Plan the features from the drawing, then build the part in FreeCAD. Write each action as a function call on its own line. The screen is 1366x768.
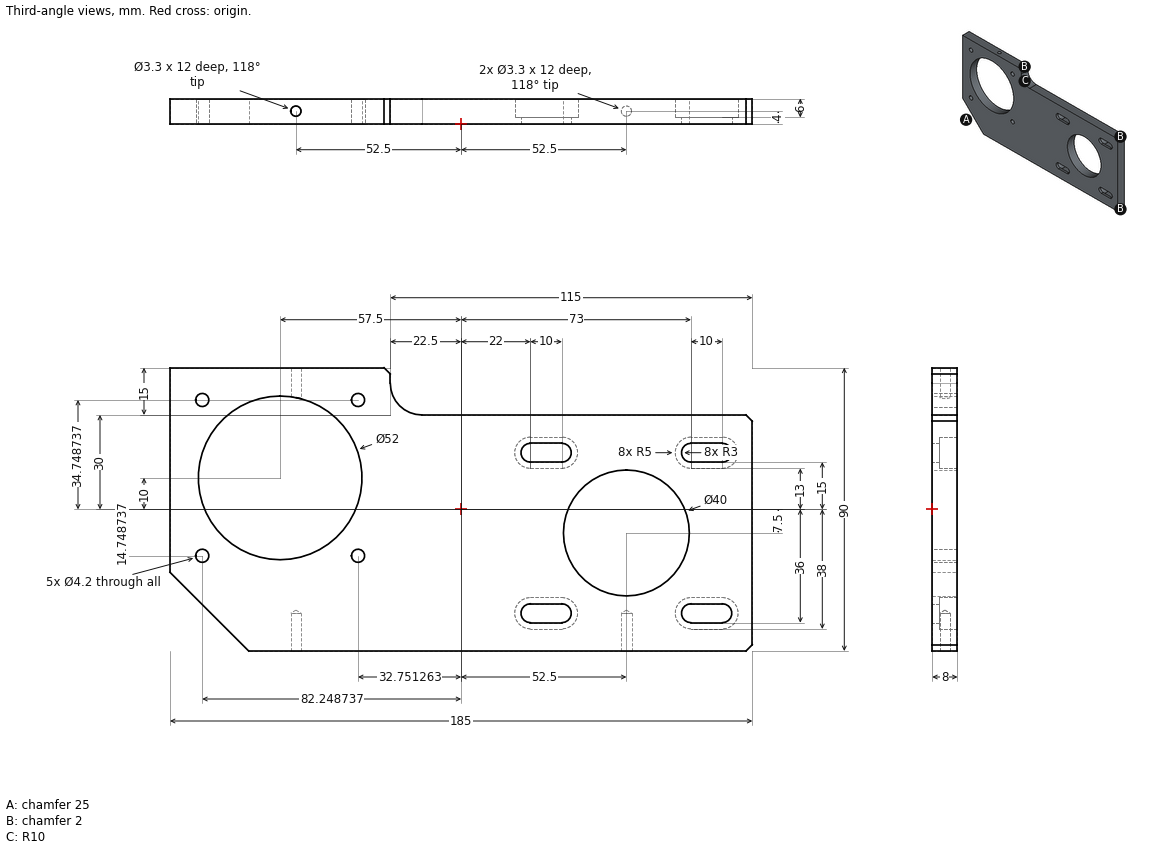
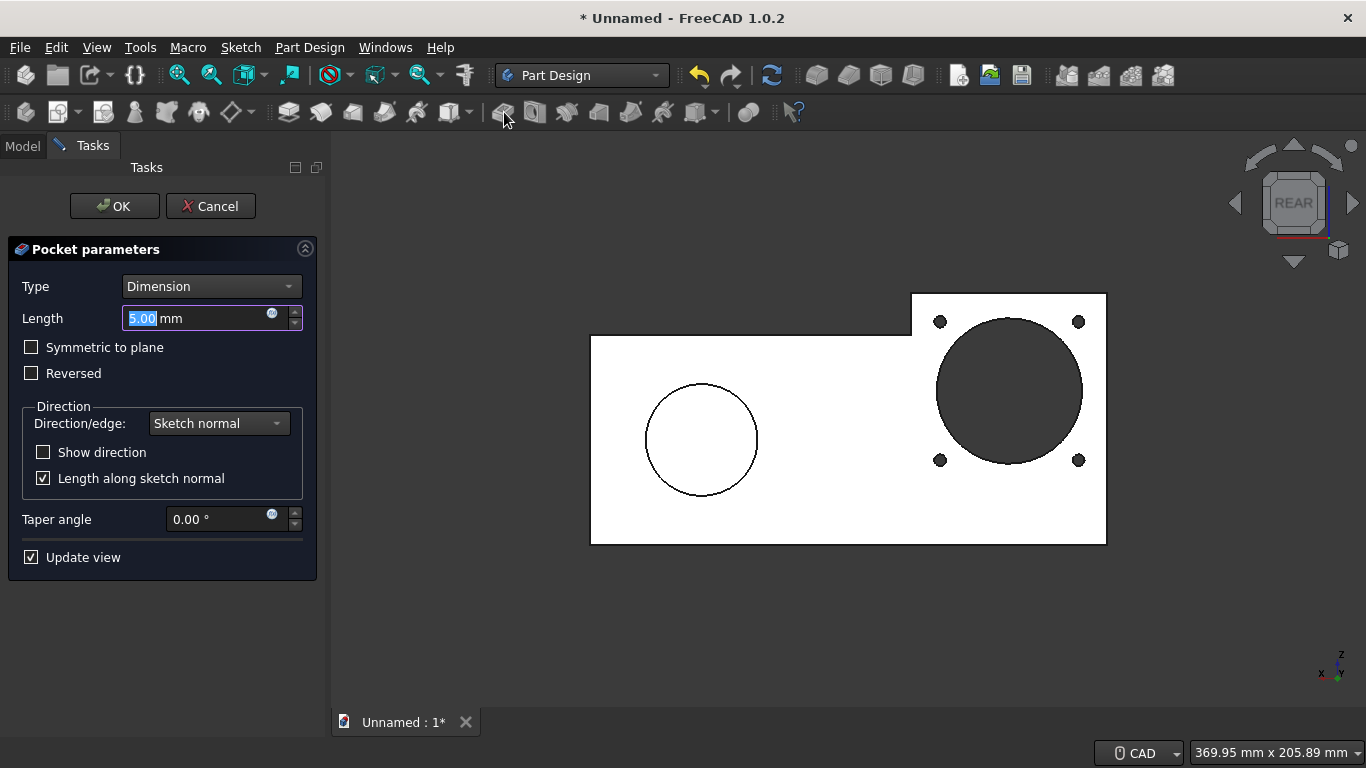
click(212, 286)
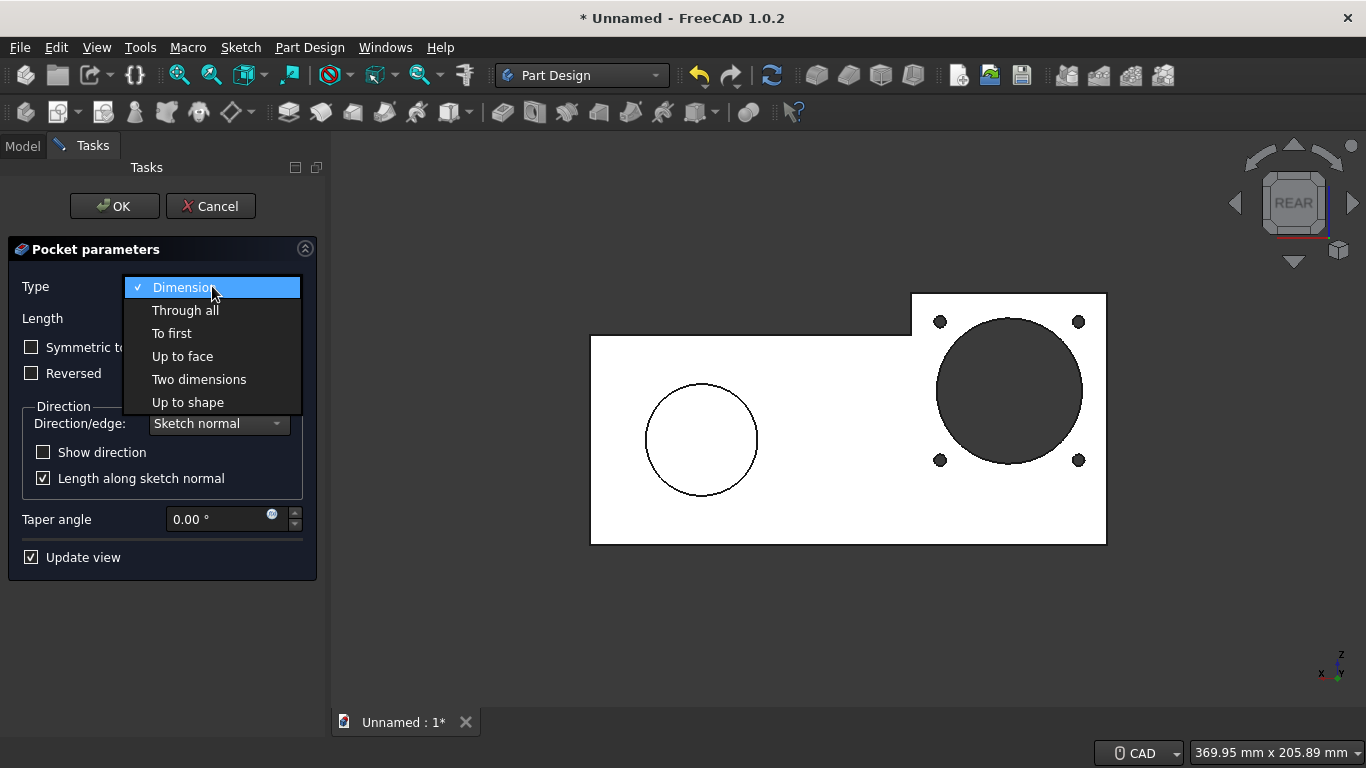
click(212, 310)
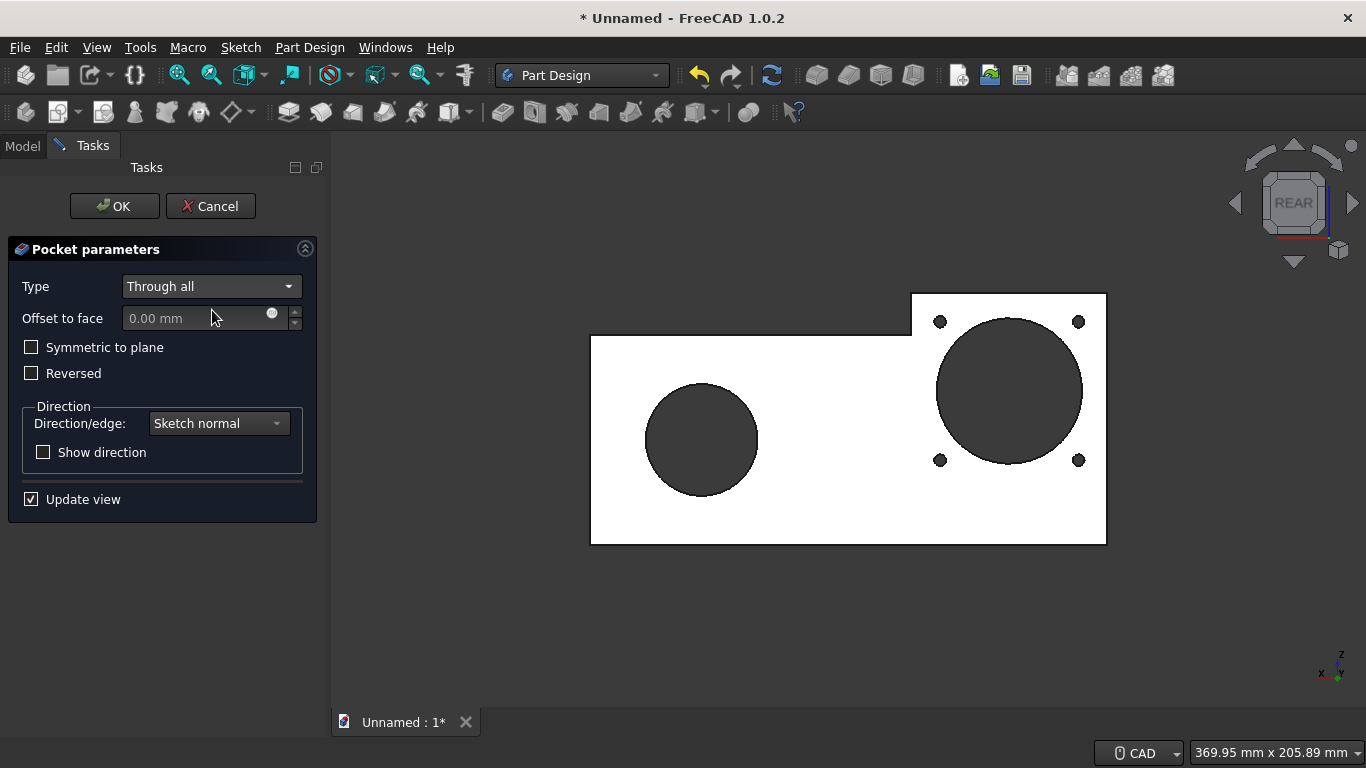
click(115, 206)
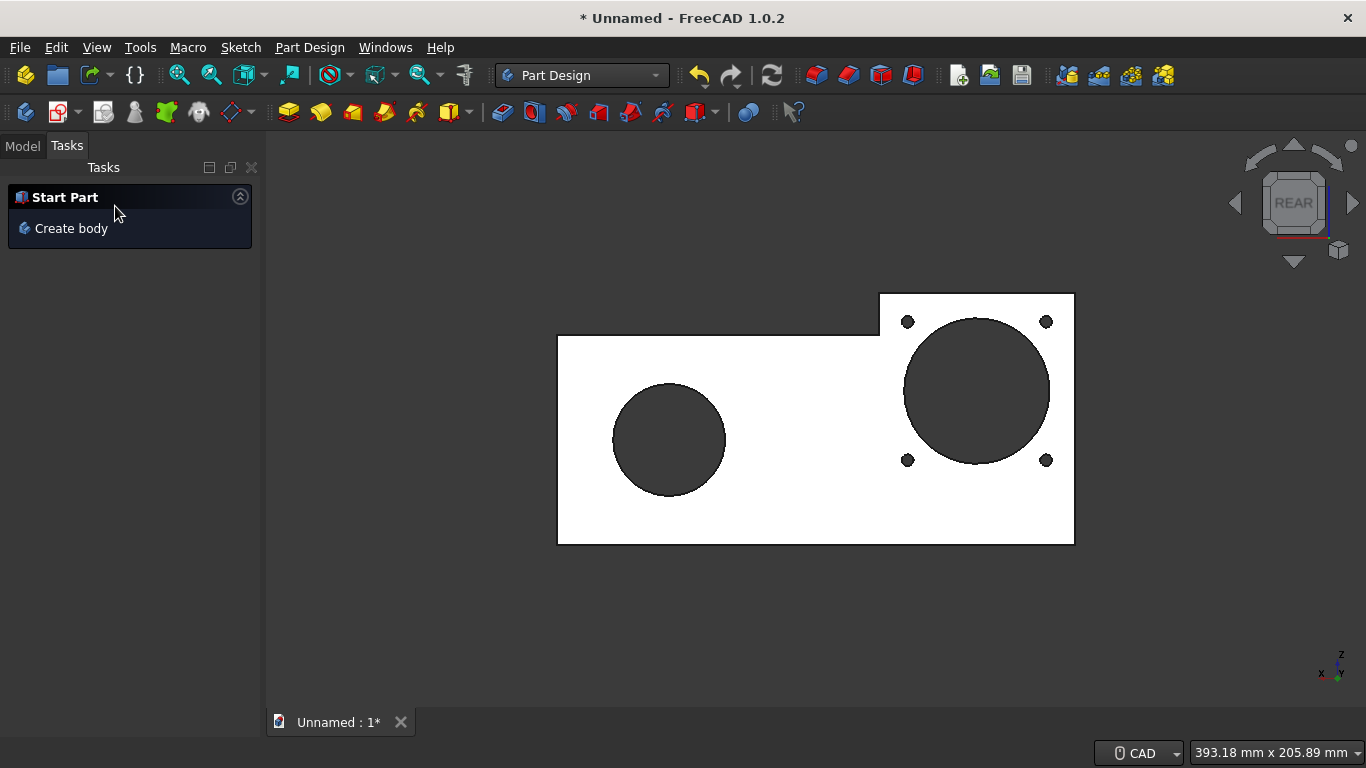
click(816, 454)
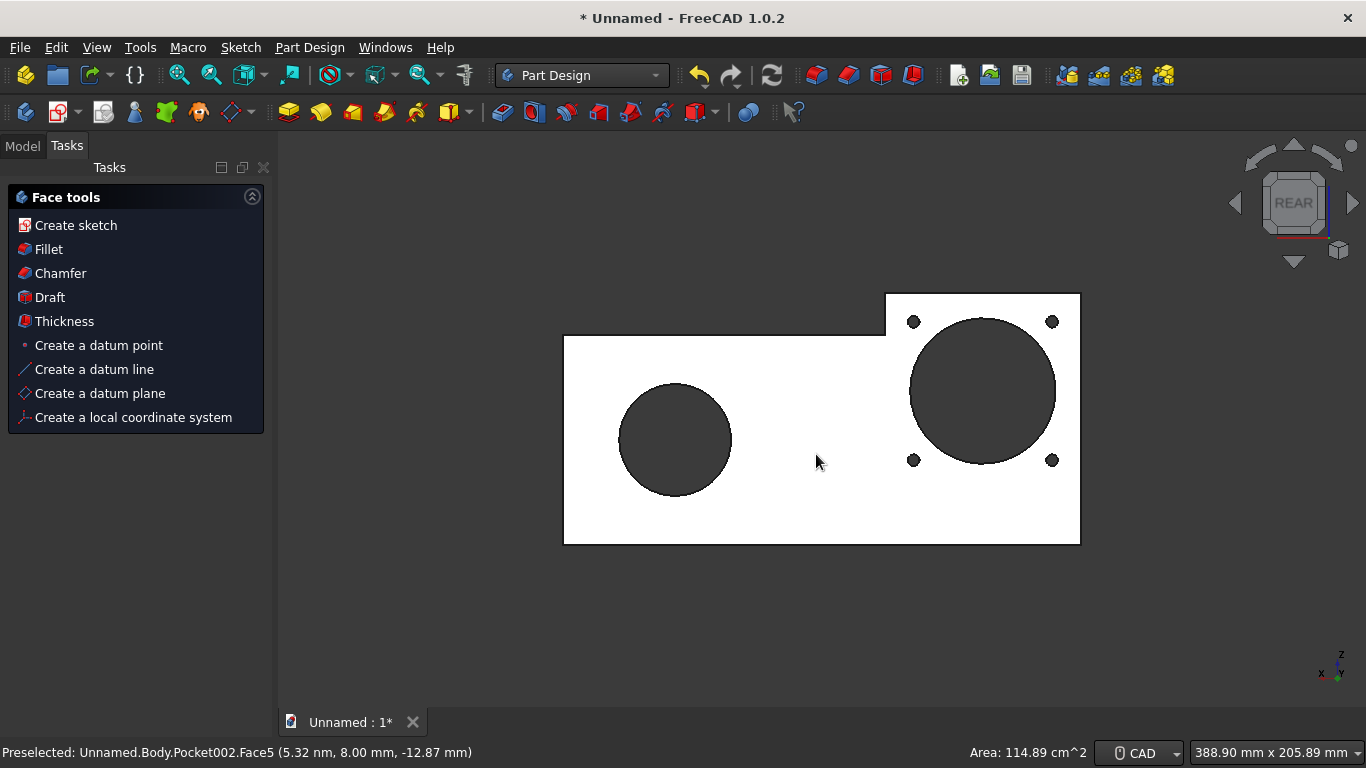
click(58, 112)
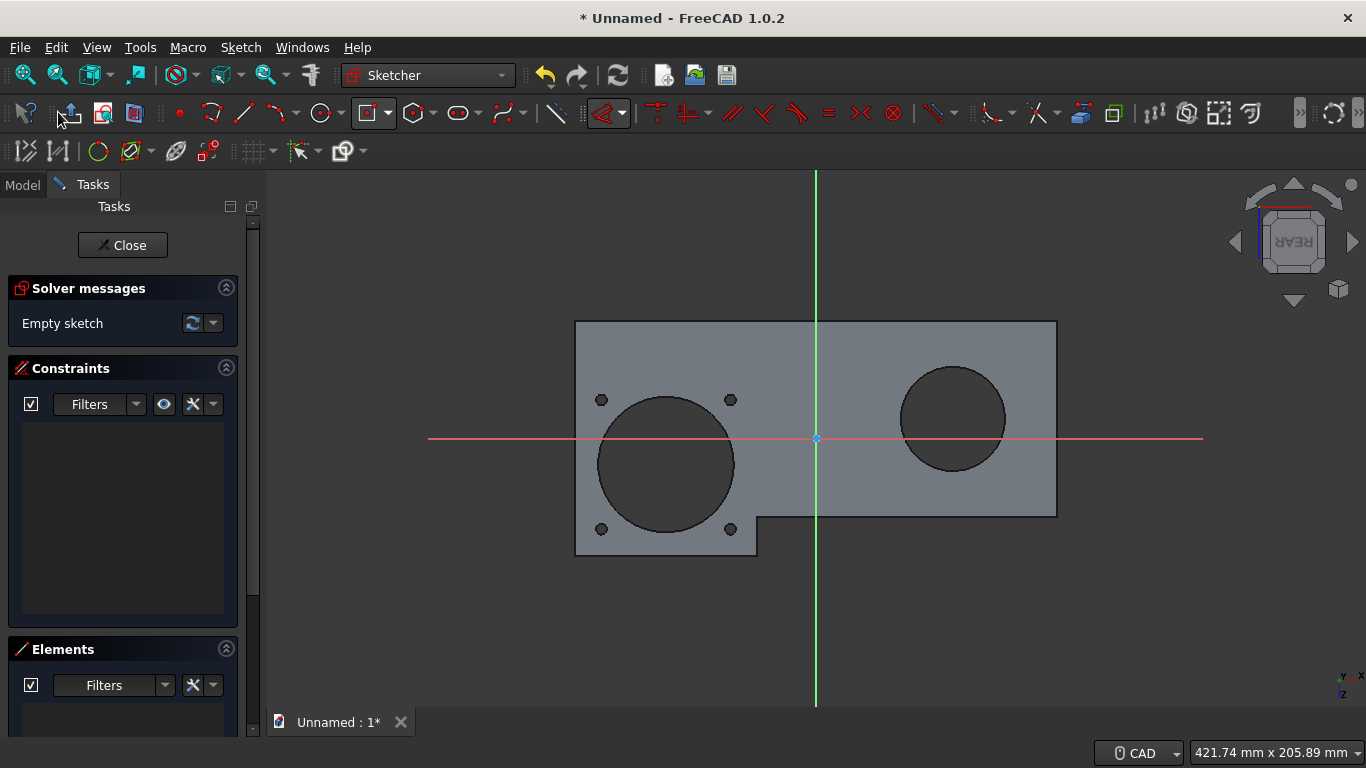
scroll(1080, 403, up, 4)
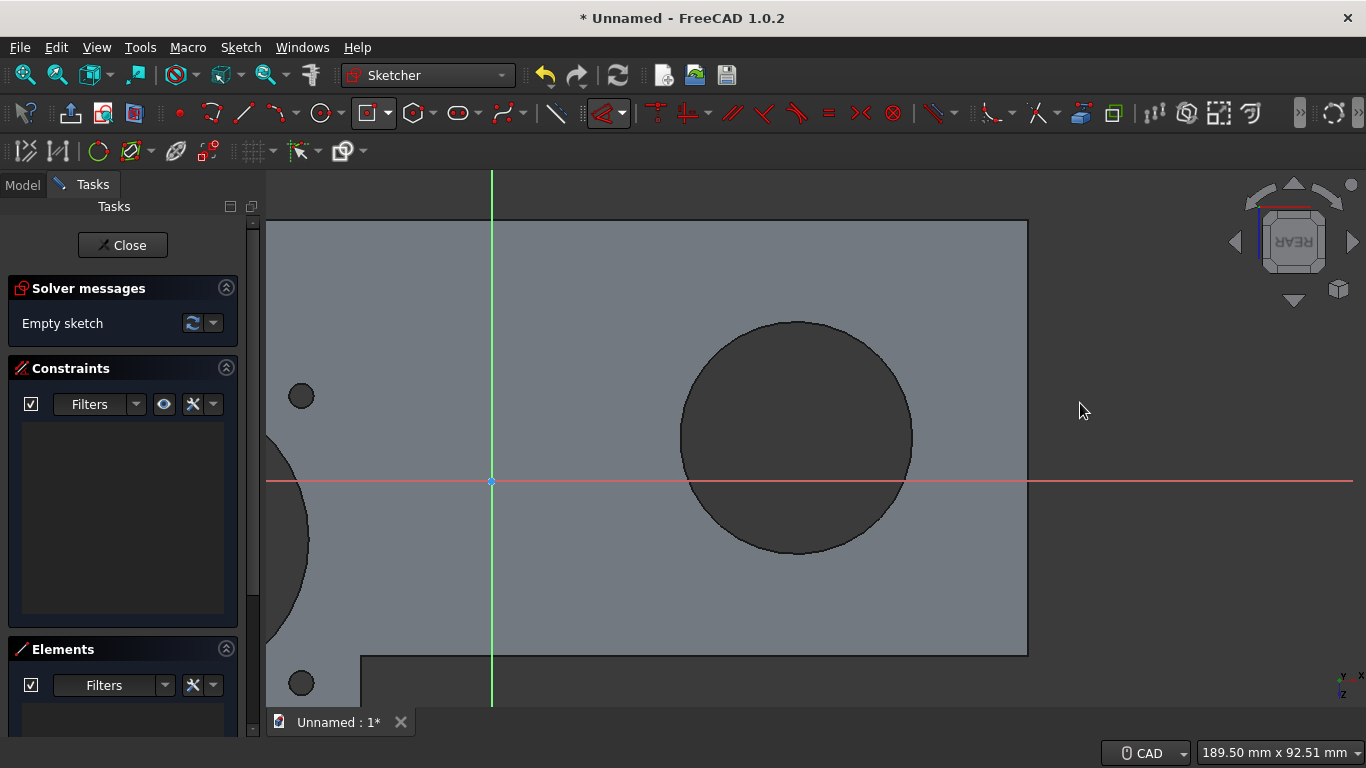
click(458, 114)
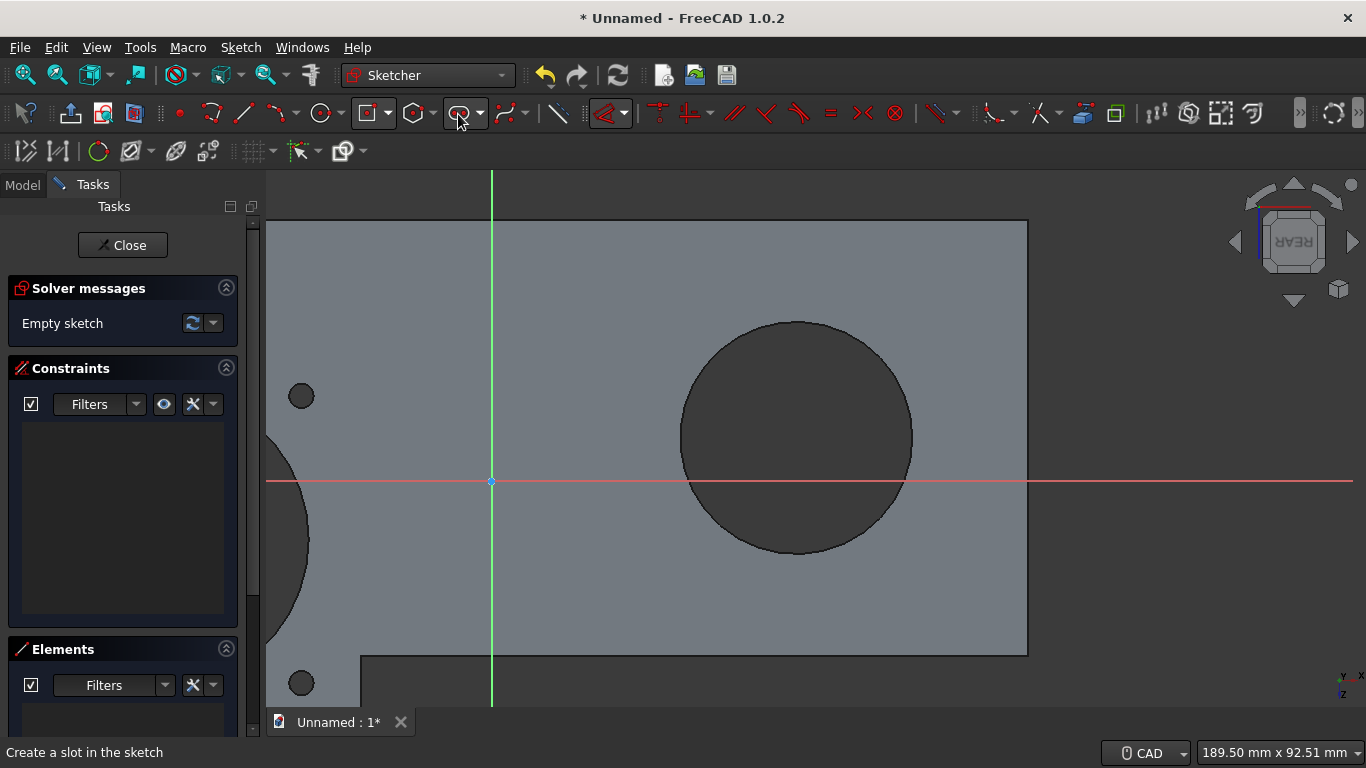
click(915, 586)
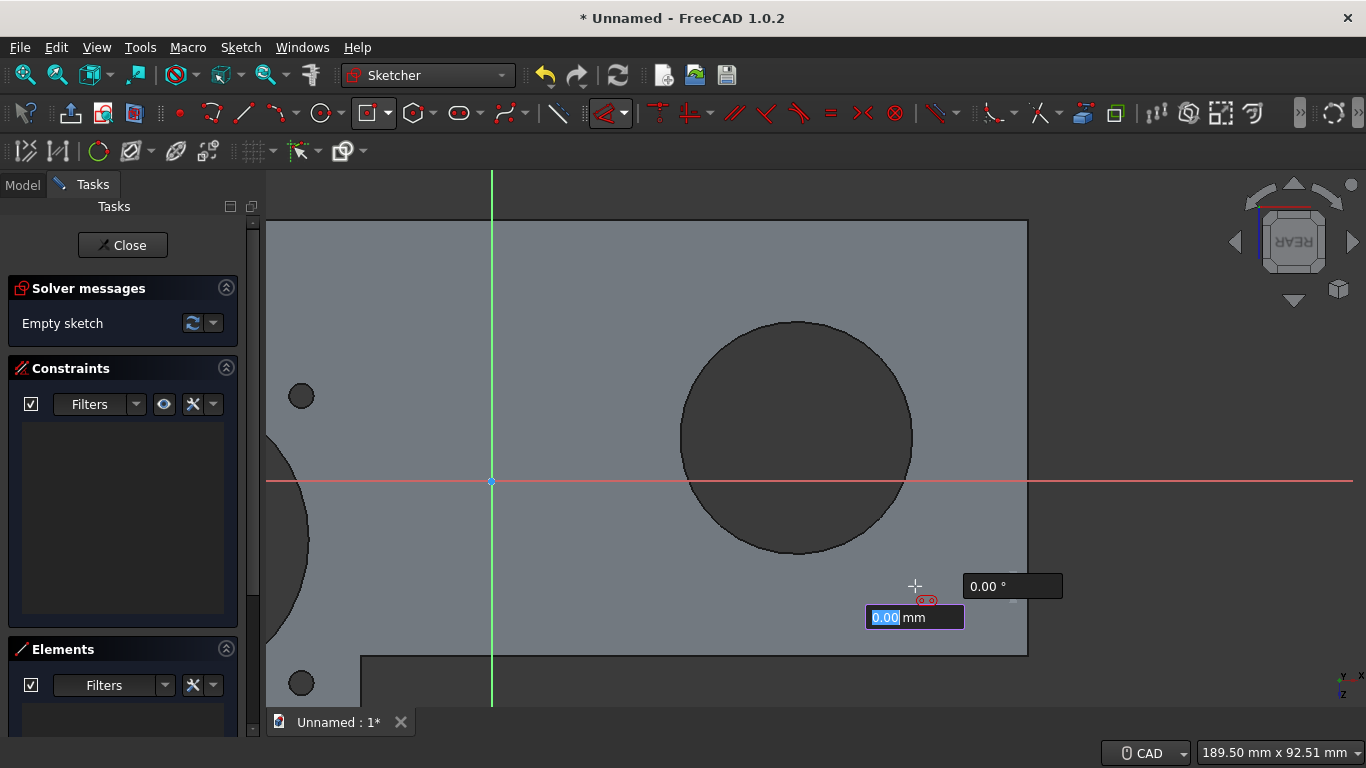
click(973, 586)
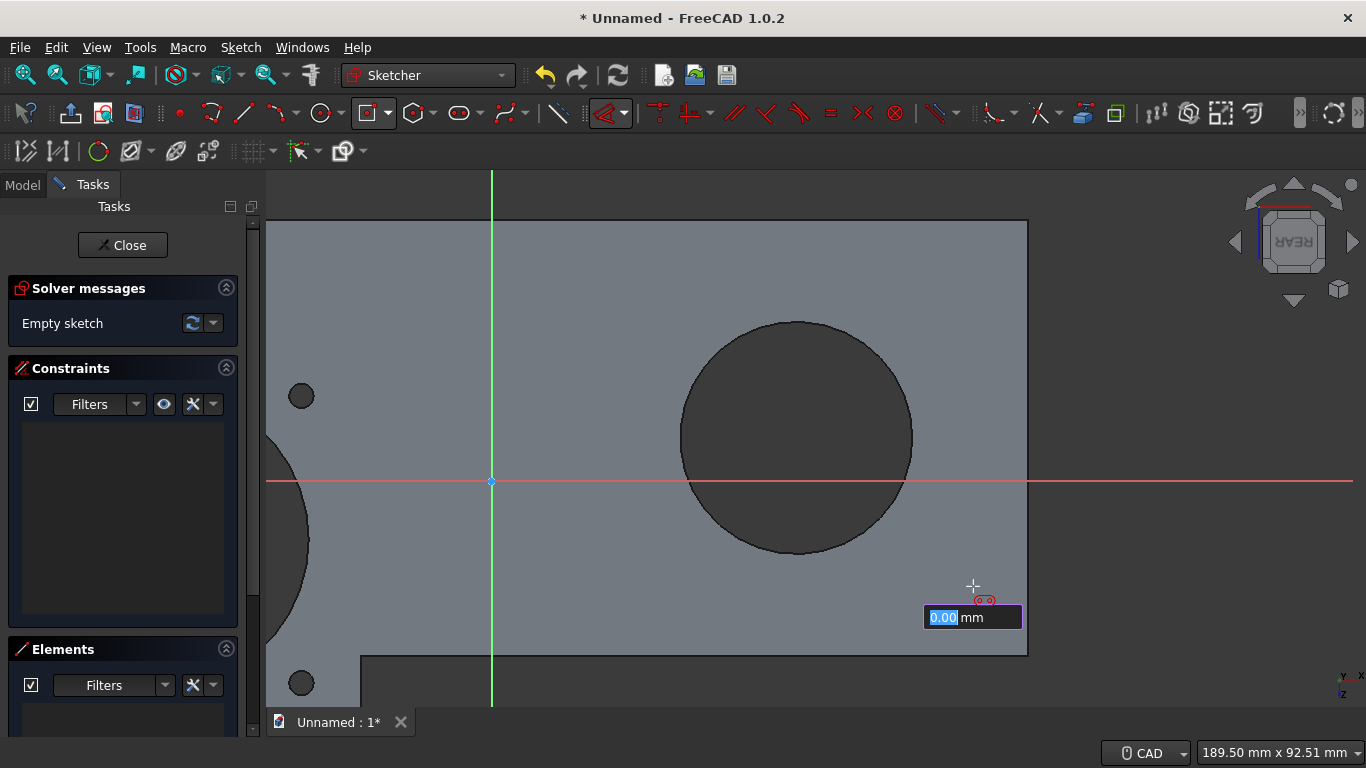
click(944, 557)